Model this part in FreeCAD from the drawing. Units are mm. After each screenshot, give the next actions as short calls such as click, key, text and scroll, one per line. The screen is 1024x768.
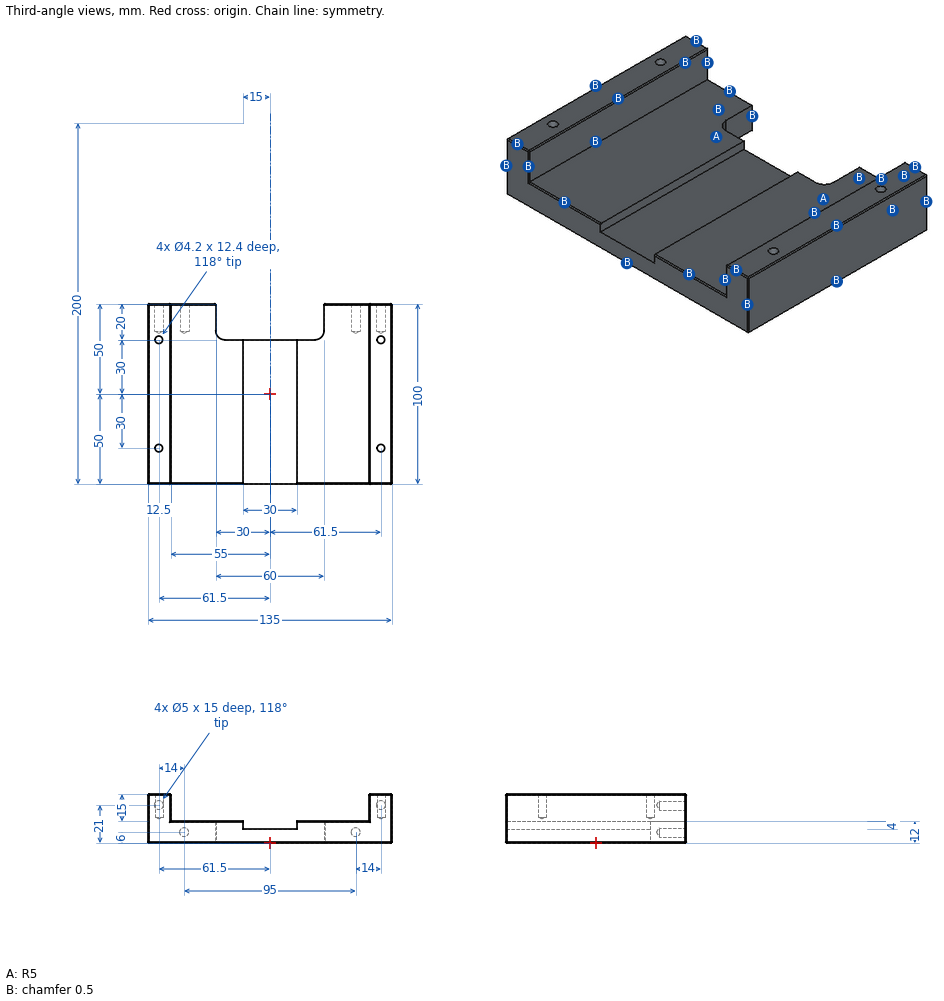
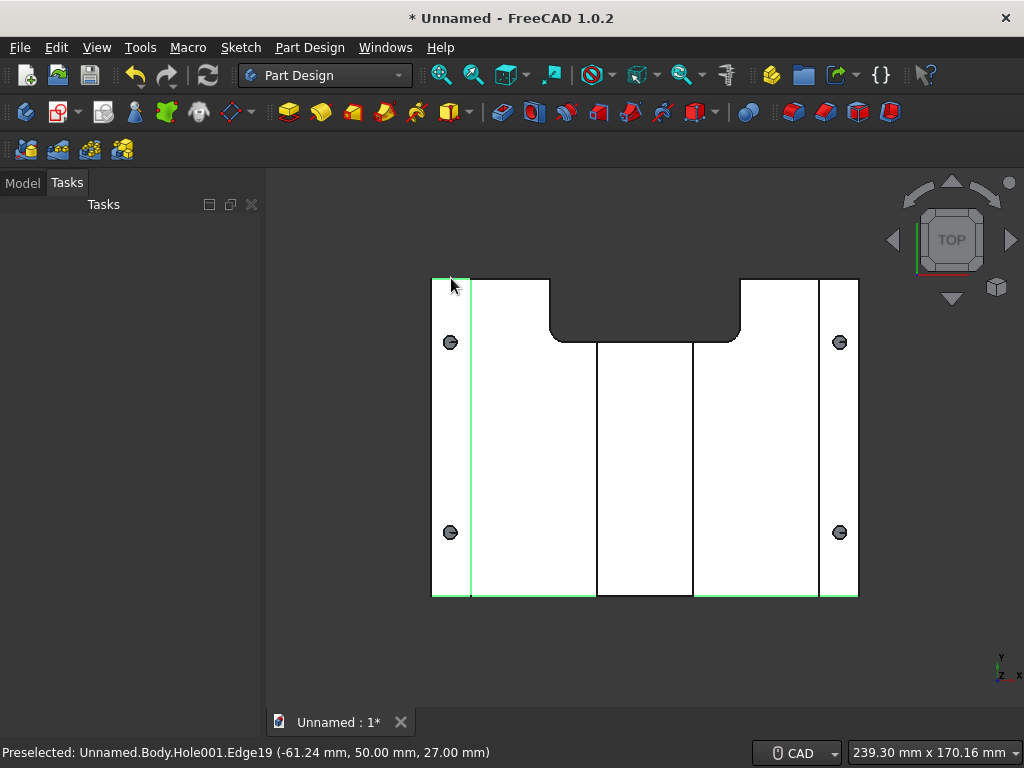
click(780, 278, ctrl)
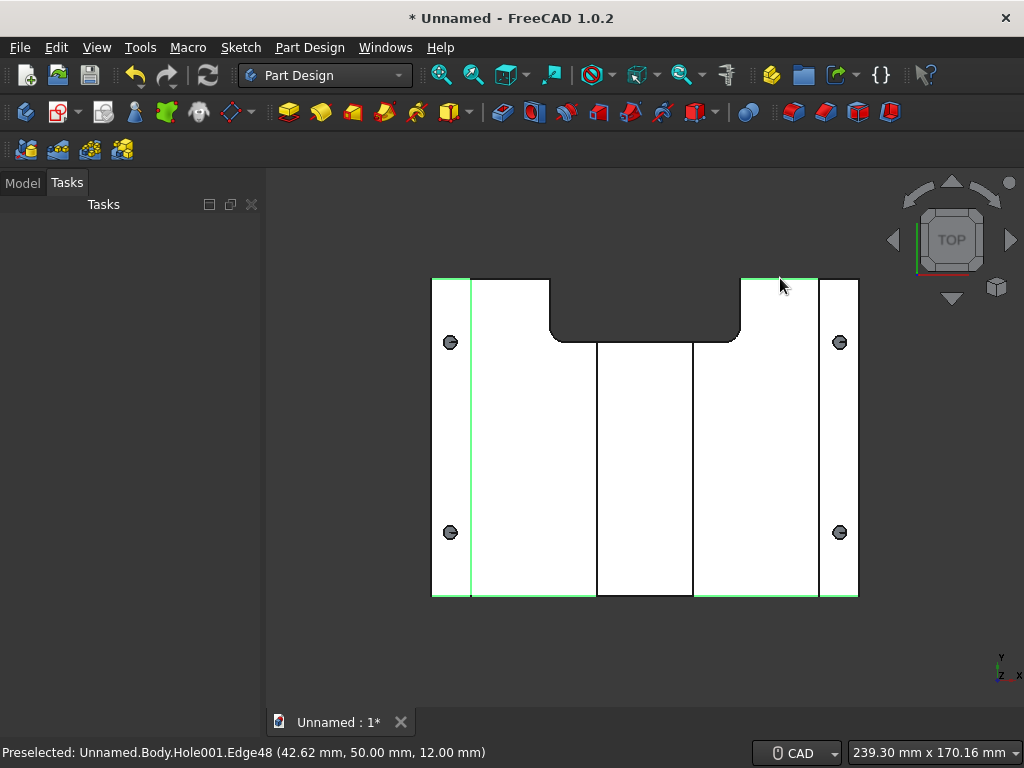
click(839, 278, ctrl)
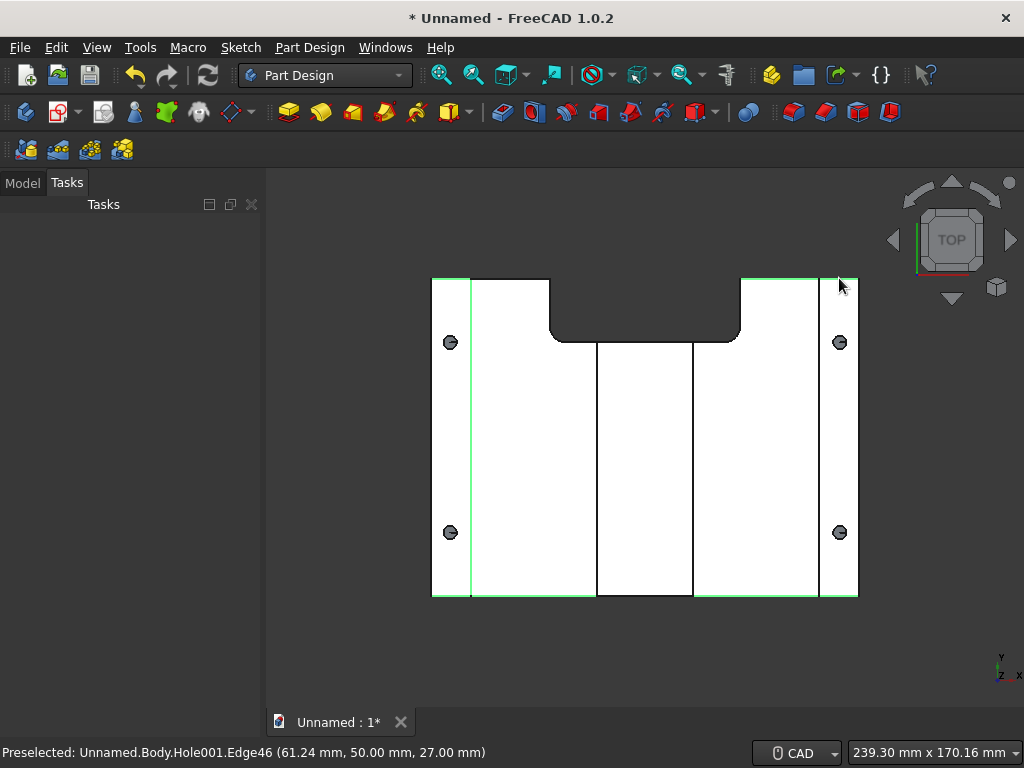
click(819, 436, ctrl)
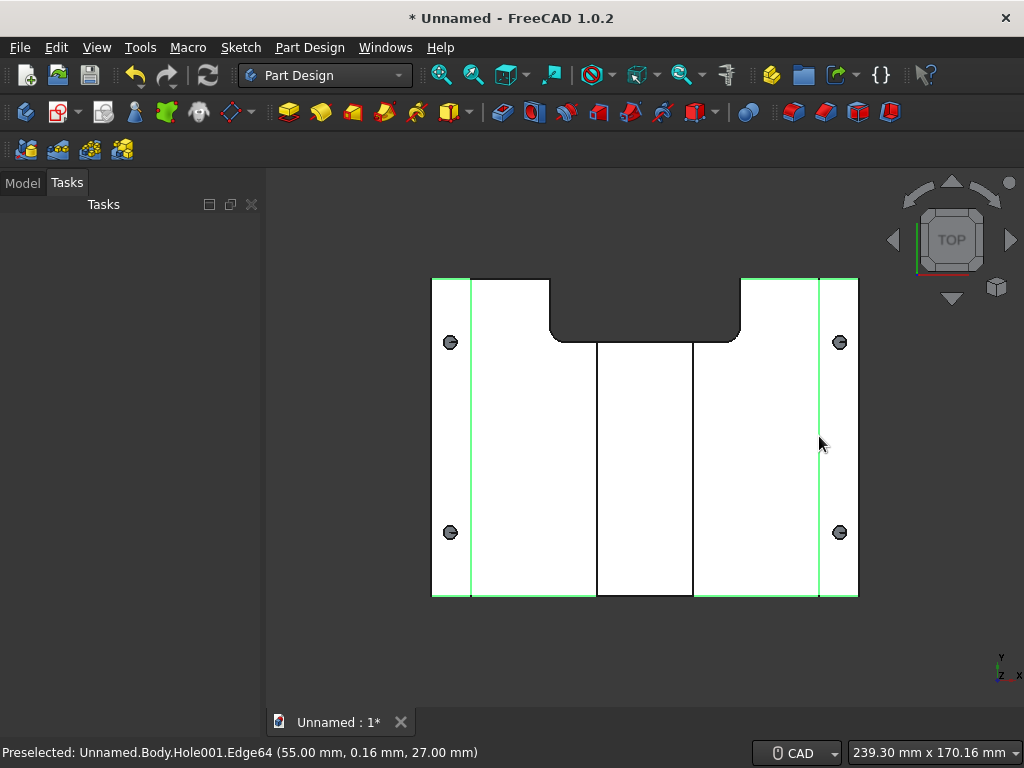
click(510, 278, ctrl)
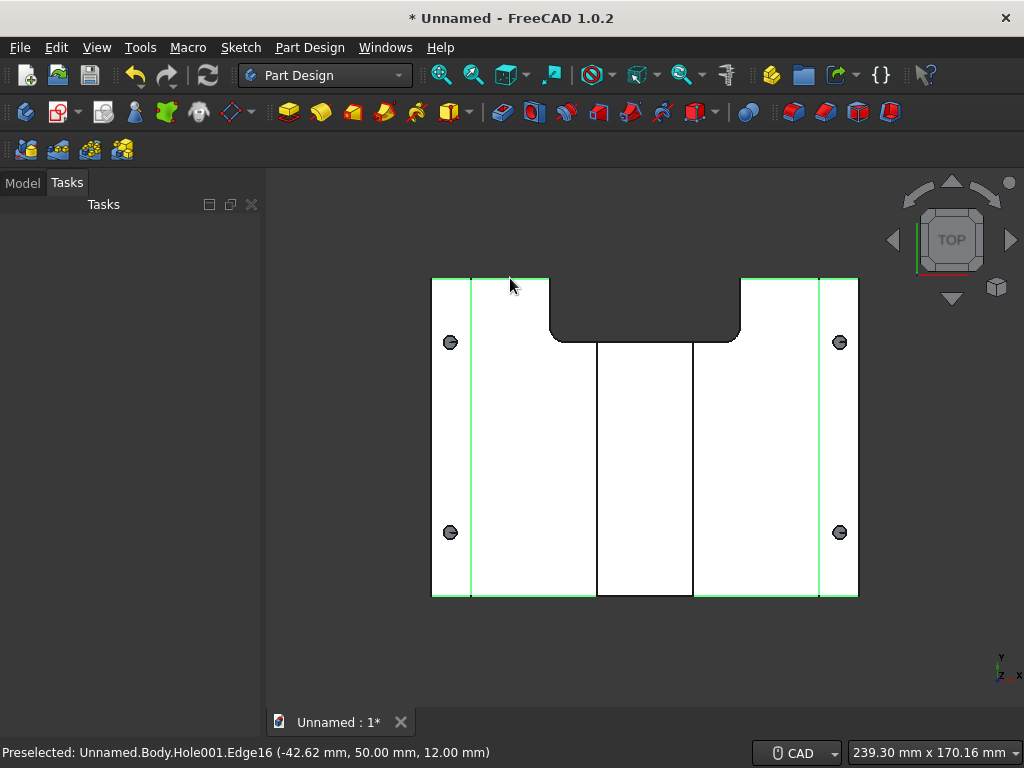
key(0)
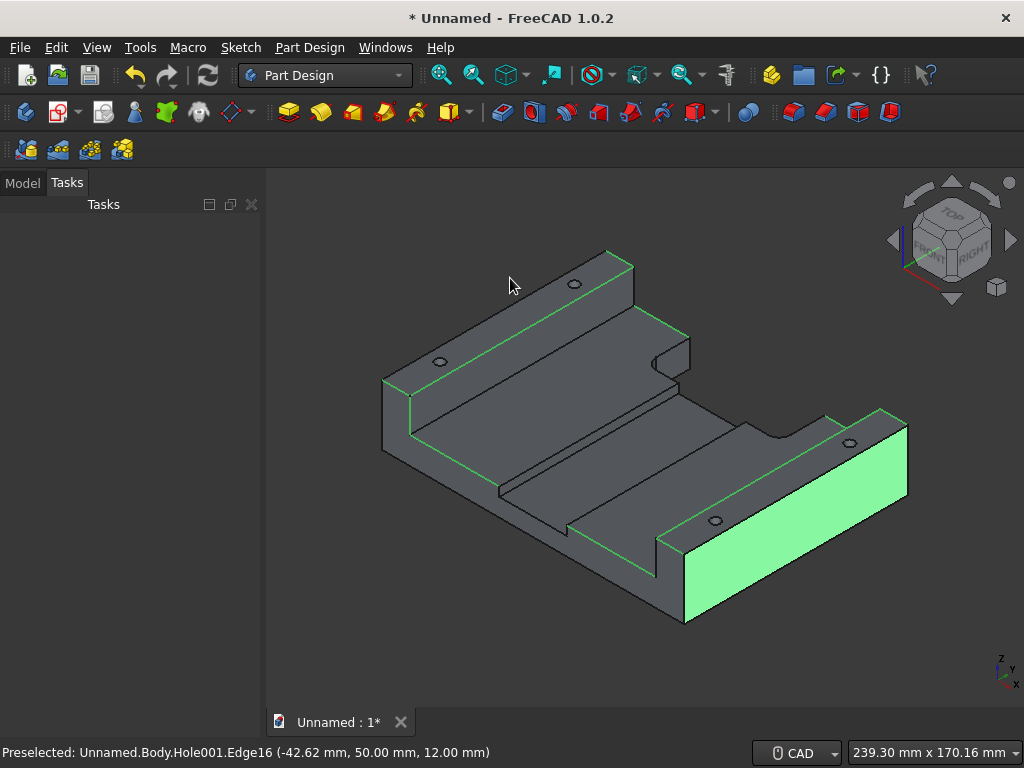
key(1)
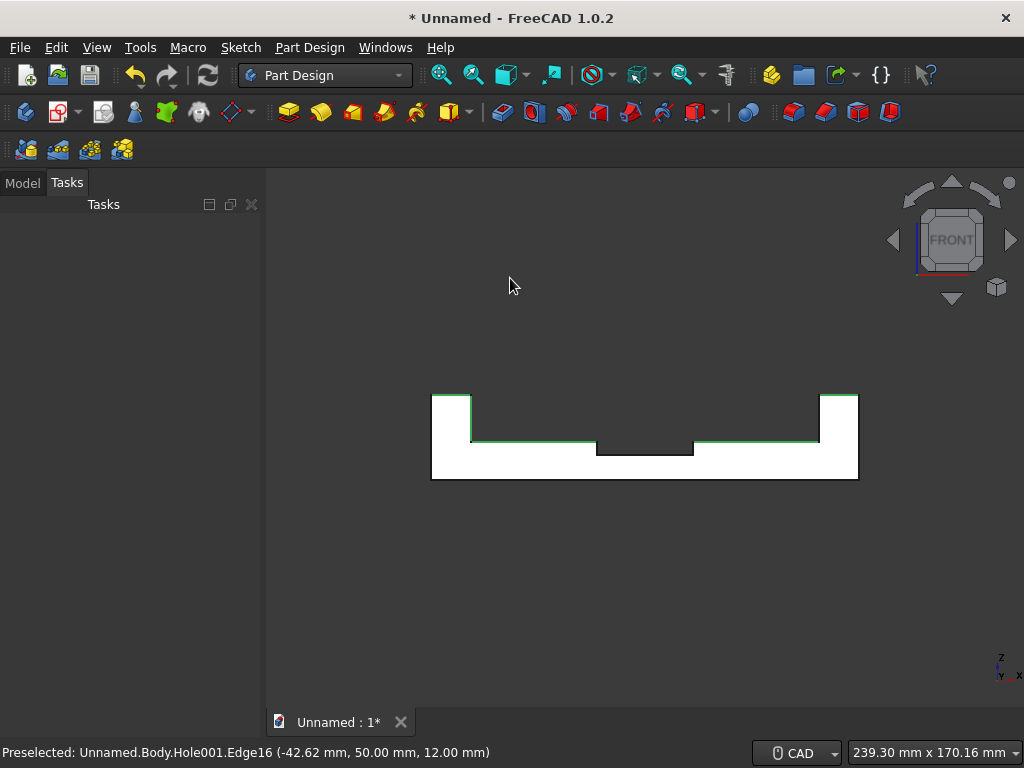
click(819, 417, ctrl)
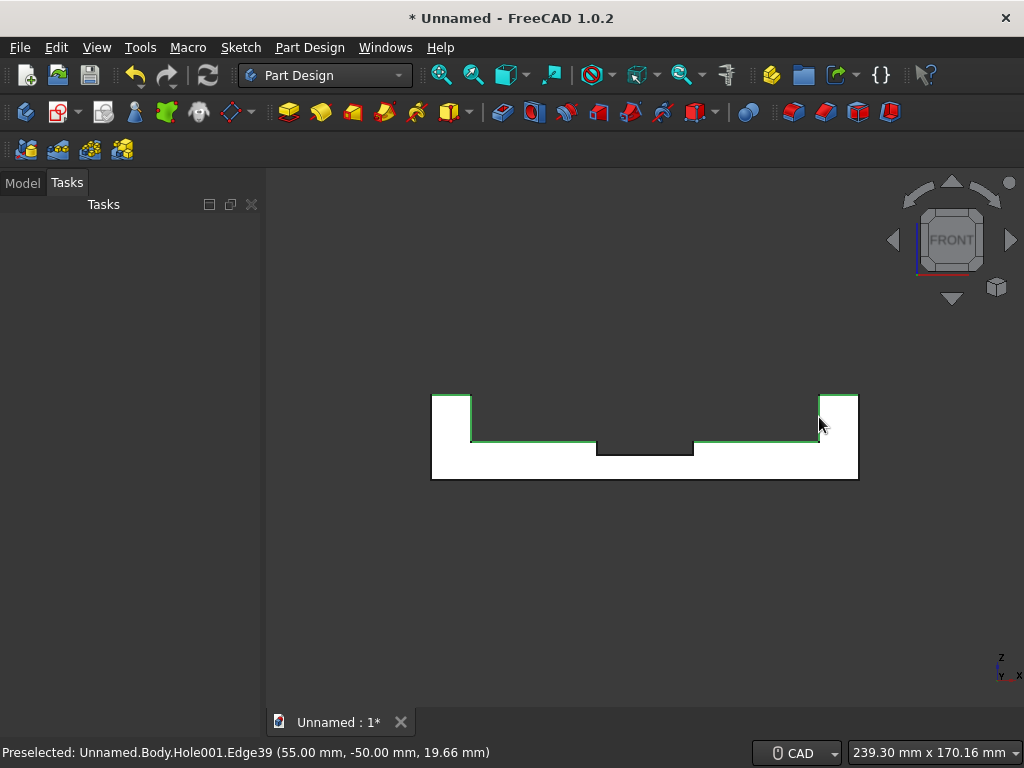
click(645, 479, ctrl)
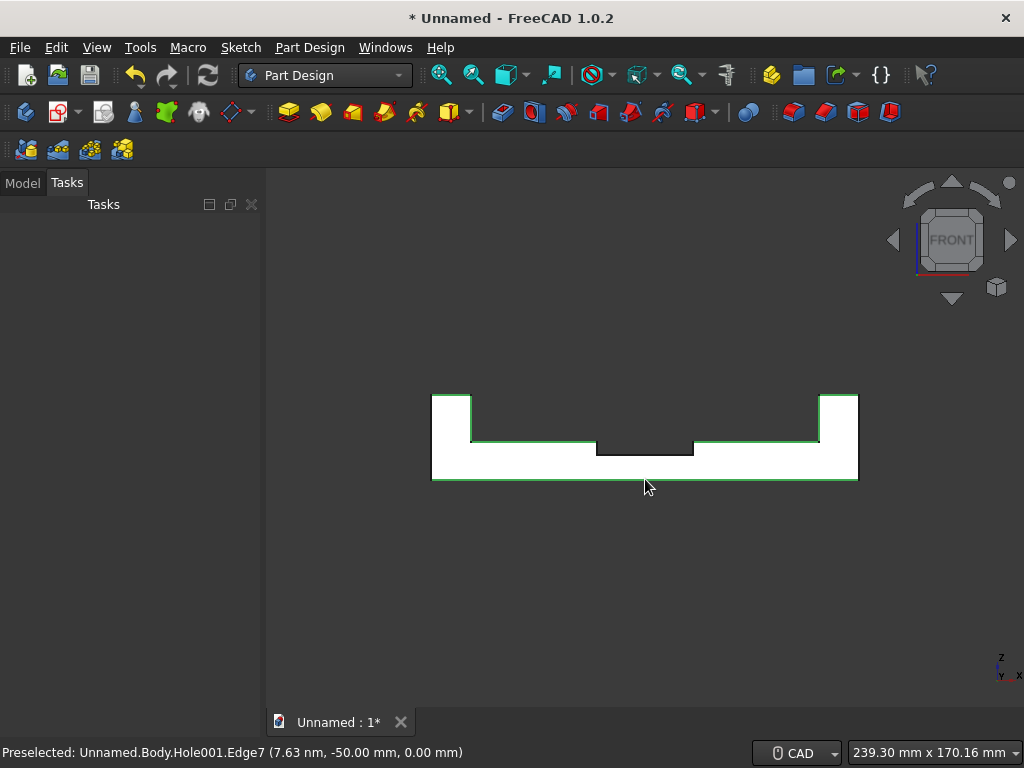
key(3)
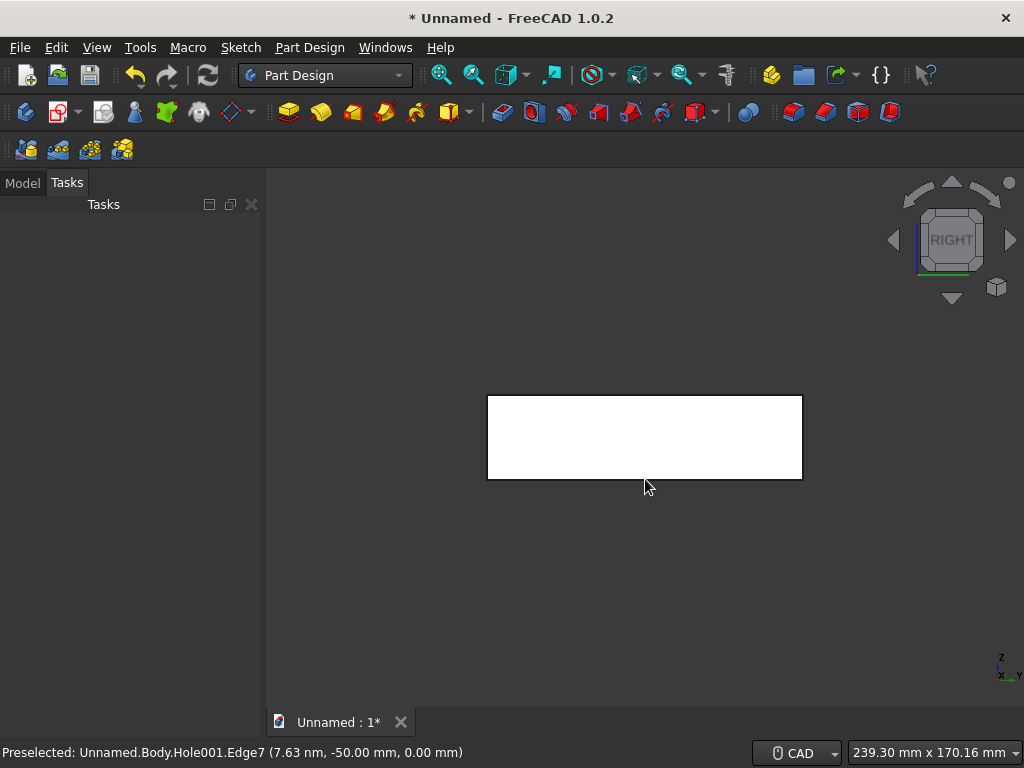
key(v)
key(f)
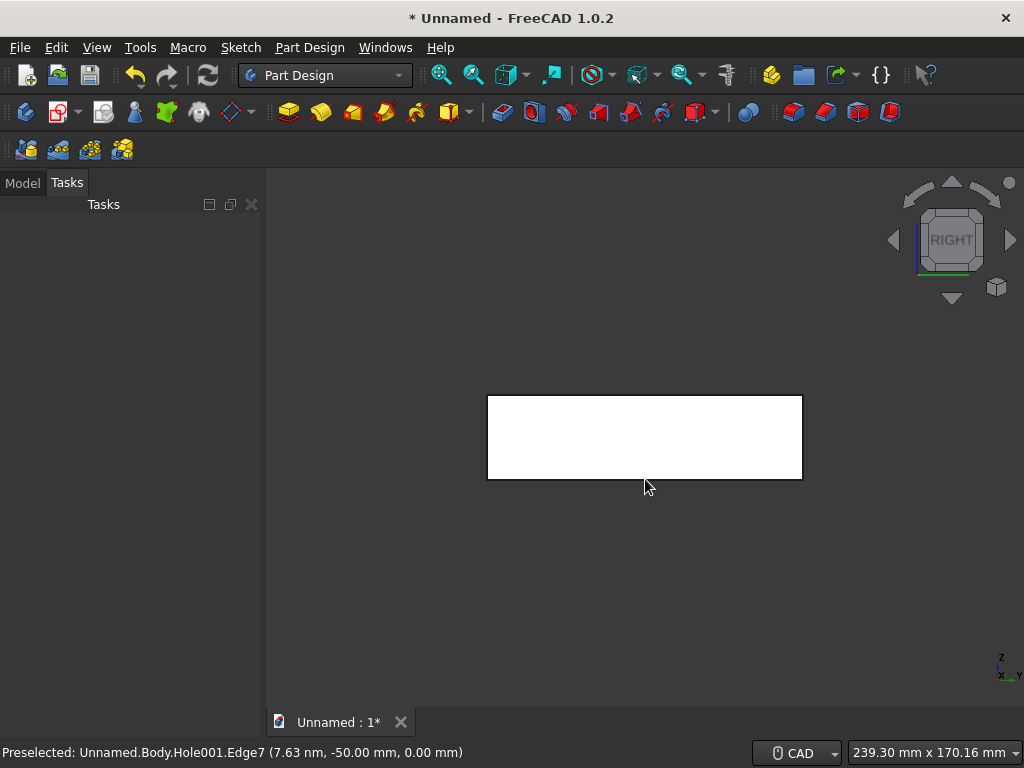
key(5)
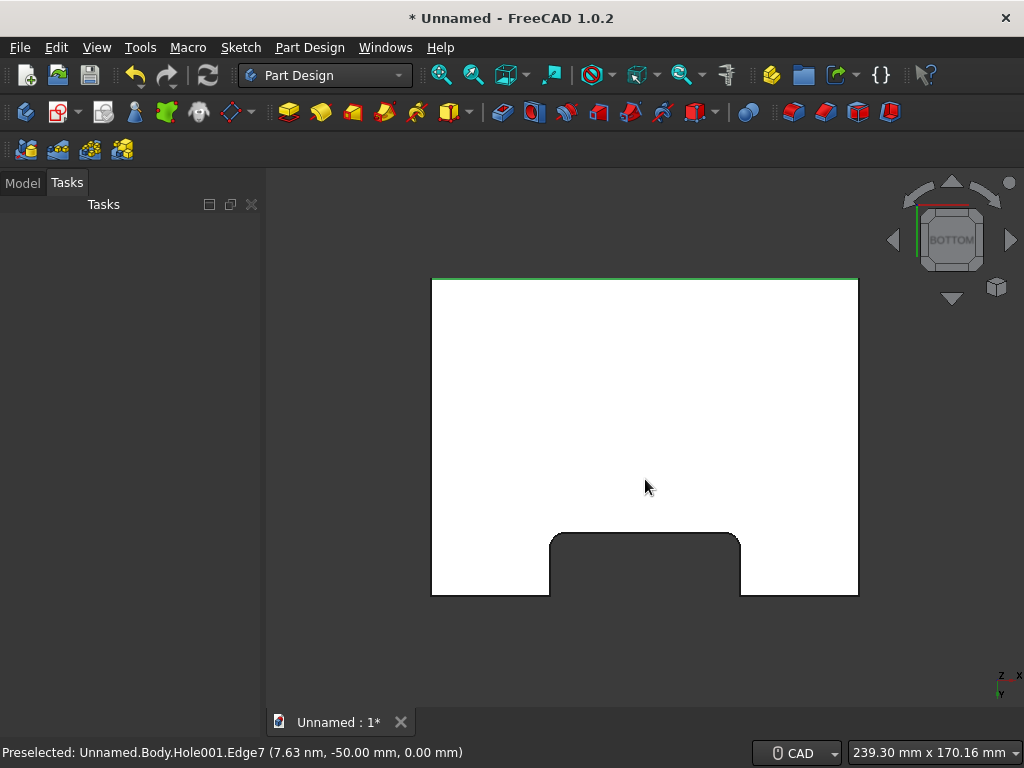
click(799, 595, ctrl)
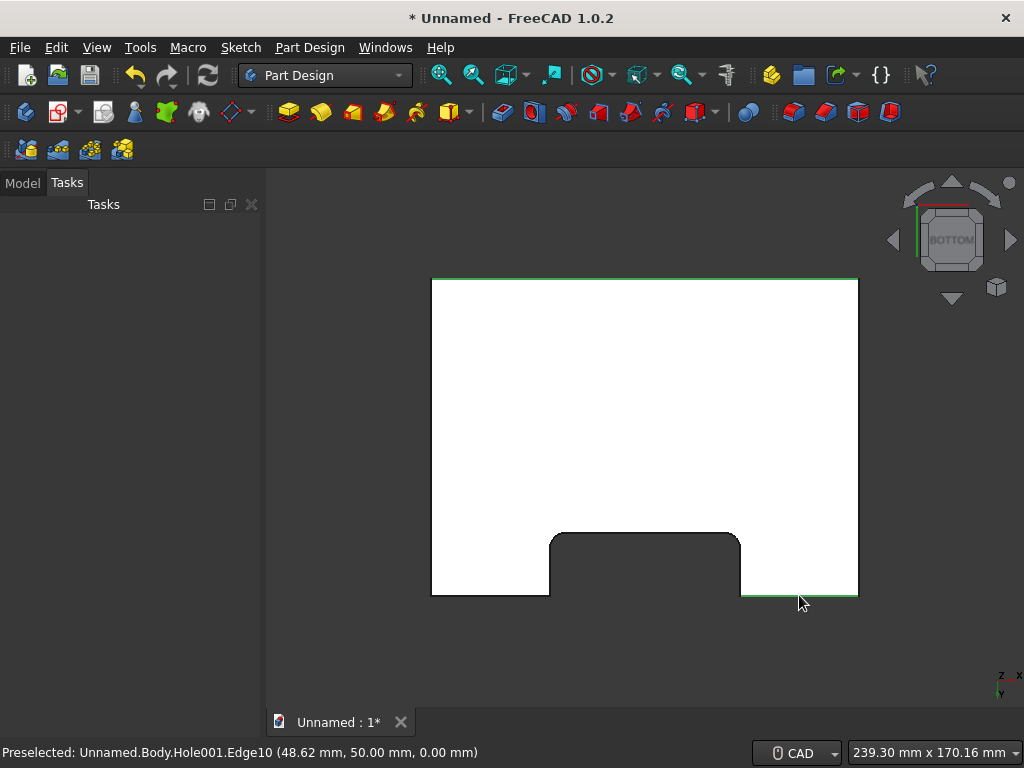
click(491, 595, ctrl)